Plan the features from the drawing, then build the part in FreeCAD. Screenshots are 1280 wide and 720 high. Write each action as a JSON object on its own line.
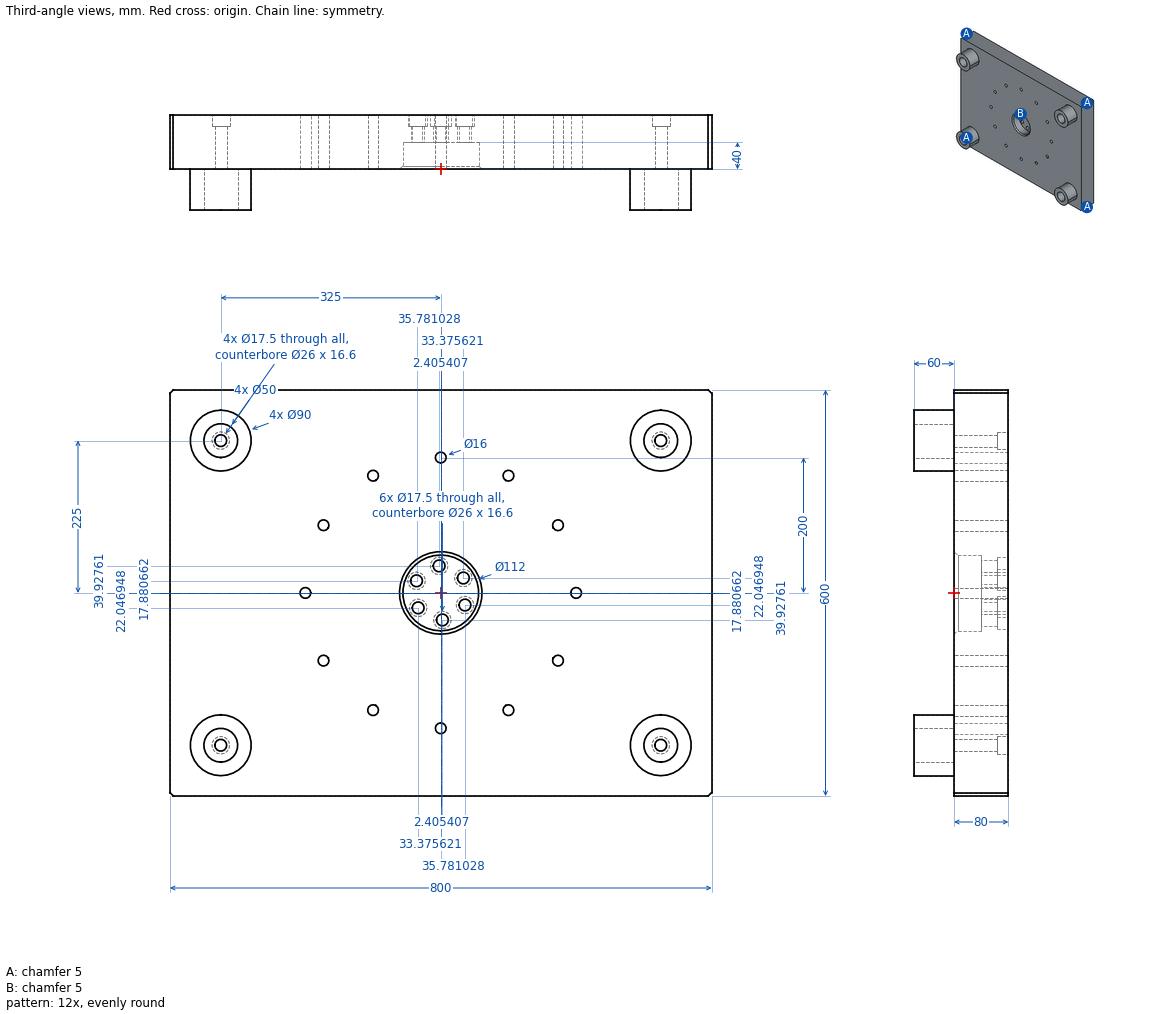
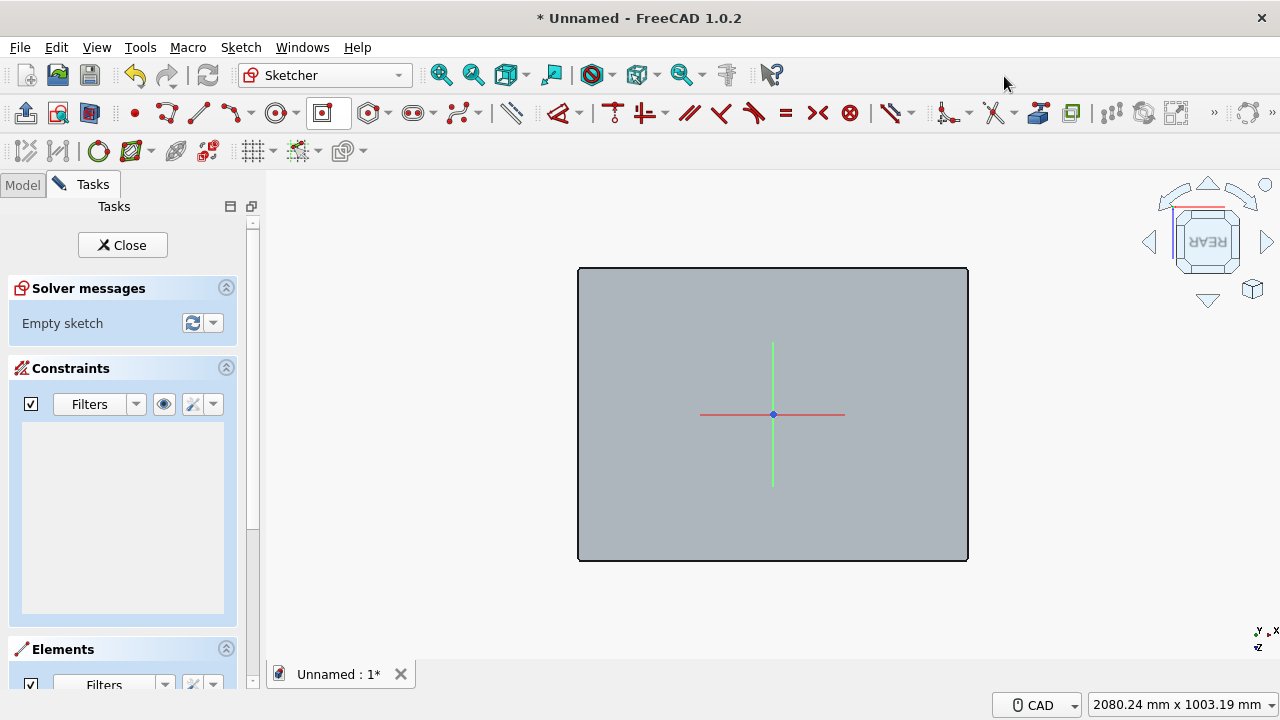
{"action": "scroll", "coordinate": [787, 415], "scroll_direction": "up", "scroll_amount": 9}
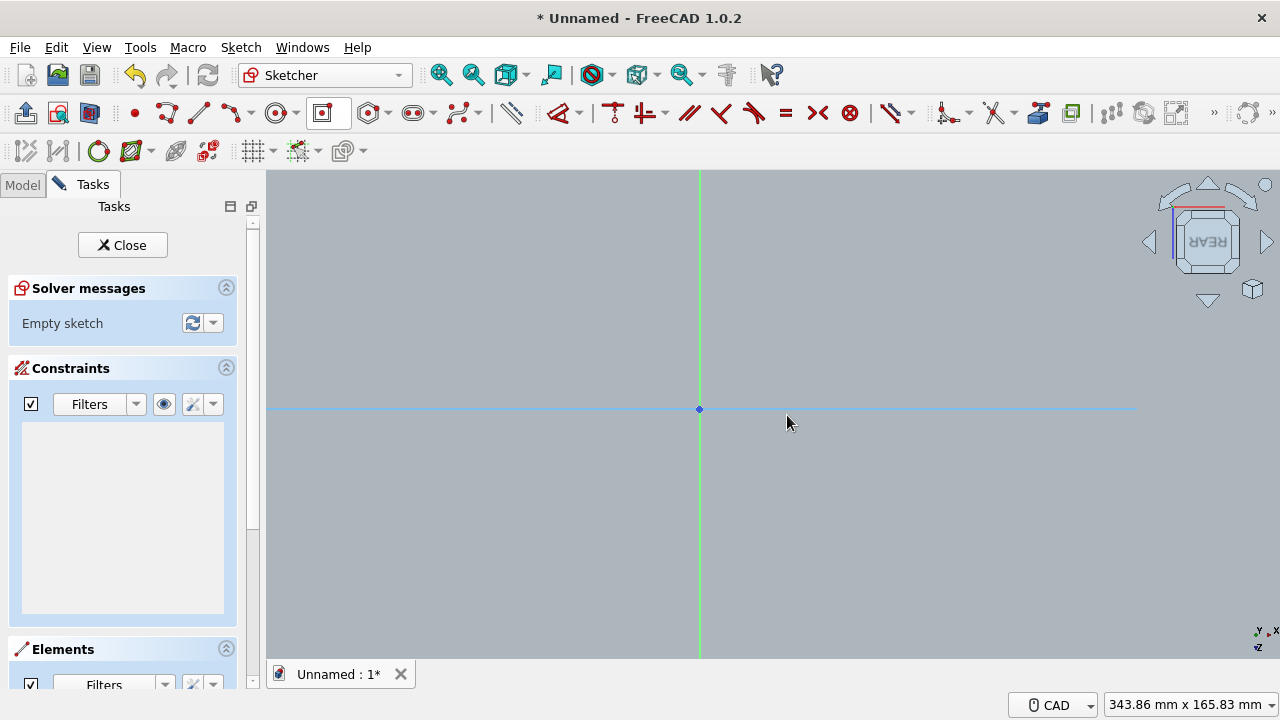
{"action": "left_click", "coordinate": [276, 114]}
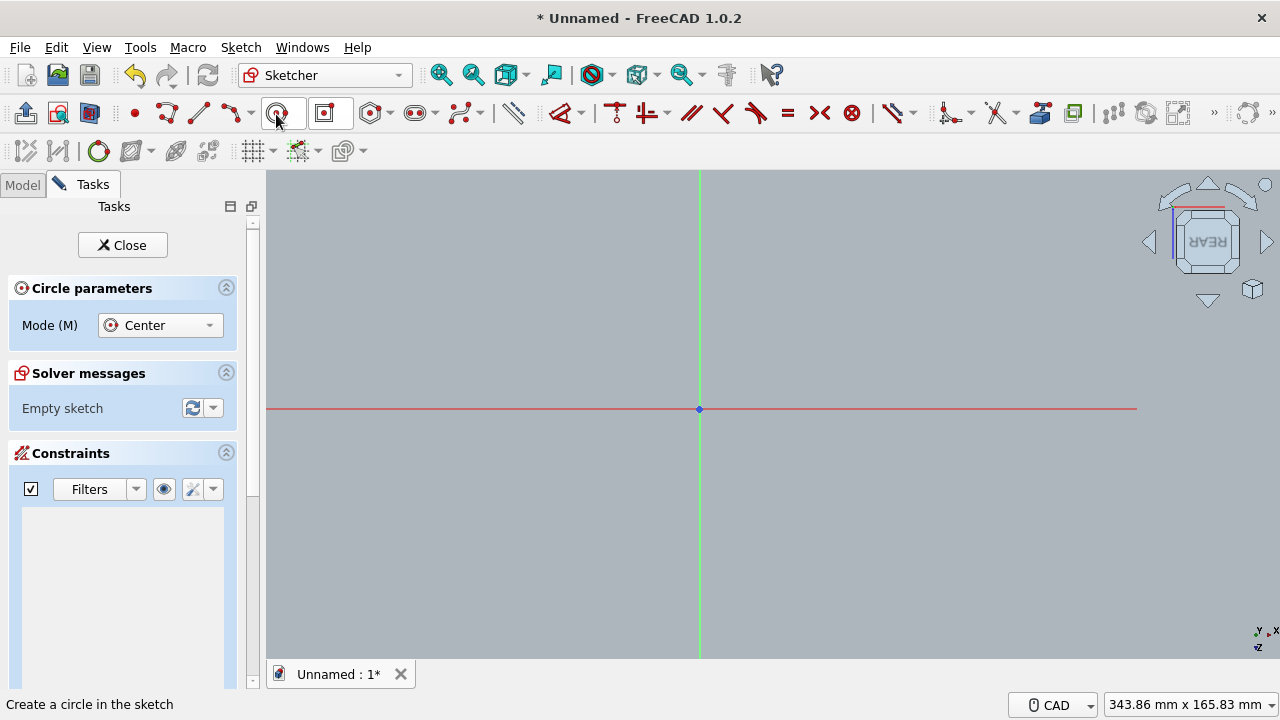
{"action": "scroll", "coordinate": [707, 292], "scroll_direction": "up", "scroll_amount": 5}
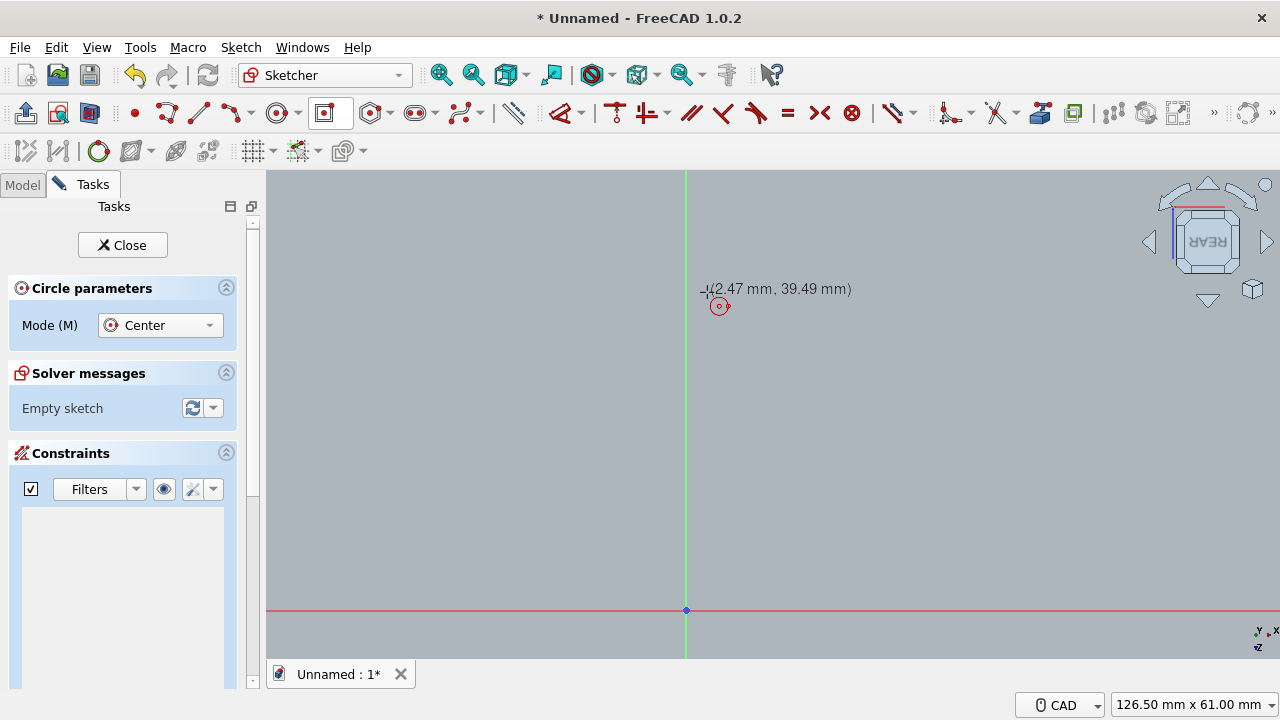
{"action": "left_click", "coordinate": [706, 291]}
{"action": "mouse_move", "coordinate": [755, 241]}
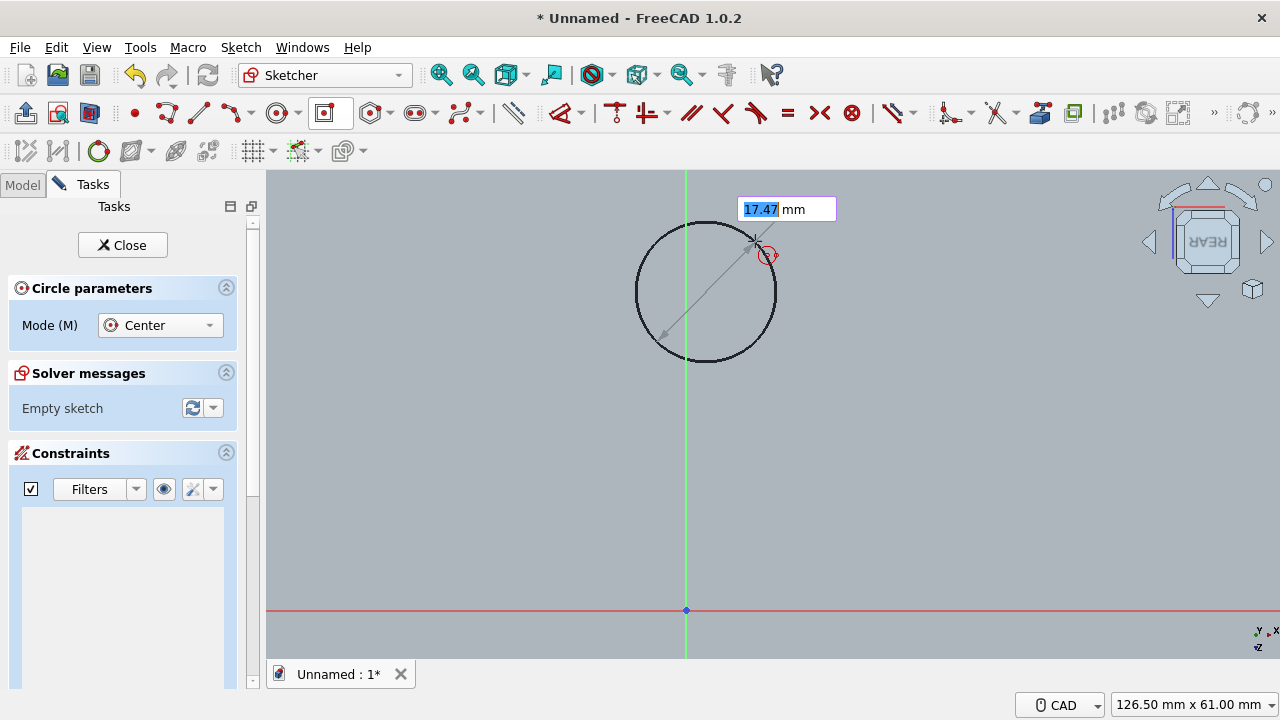
{"action": "type", "text": "17.5"}
{"action": "key", "text": "Return"}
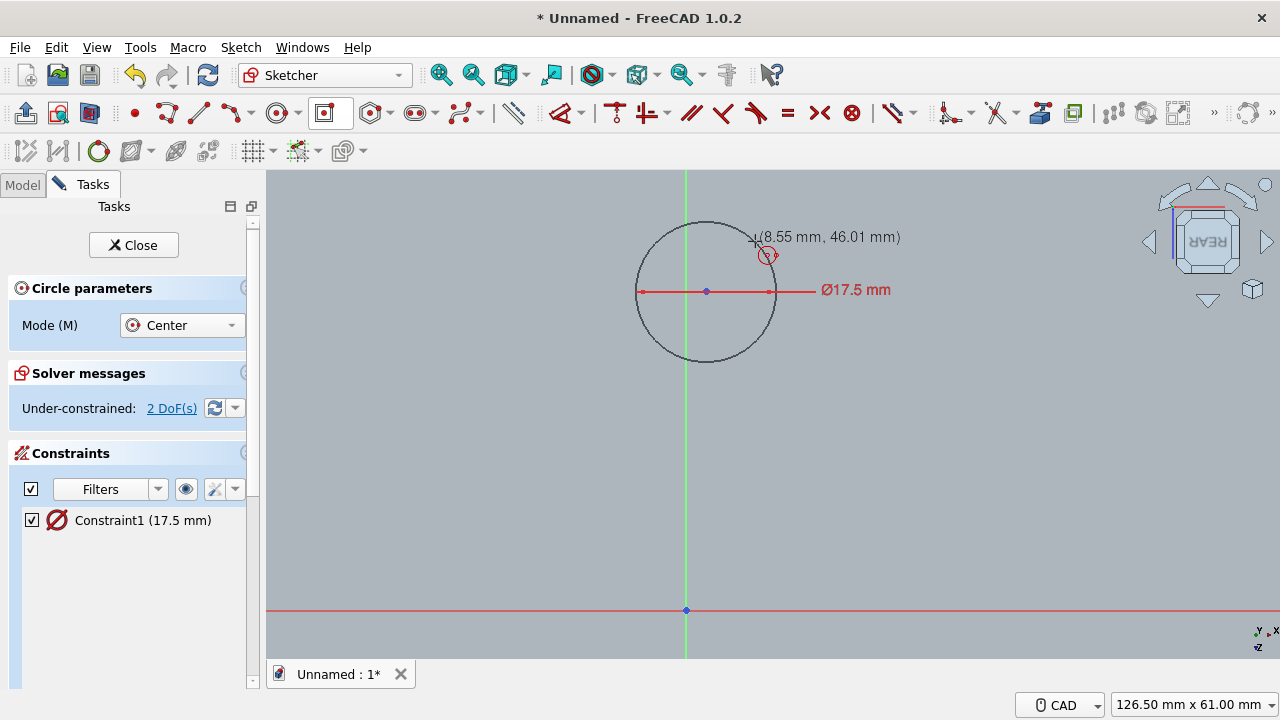
{"action": "left_click", "coordinate": [973, 467]}
{"action": "mouse_move", "coordinate": [1023, 418]}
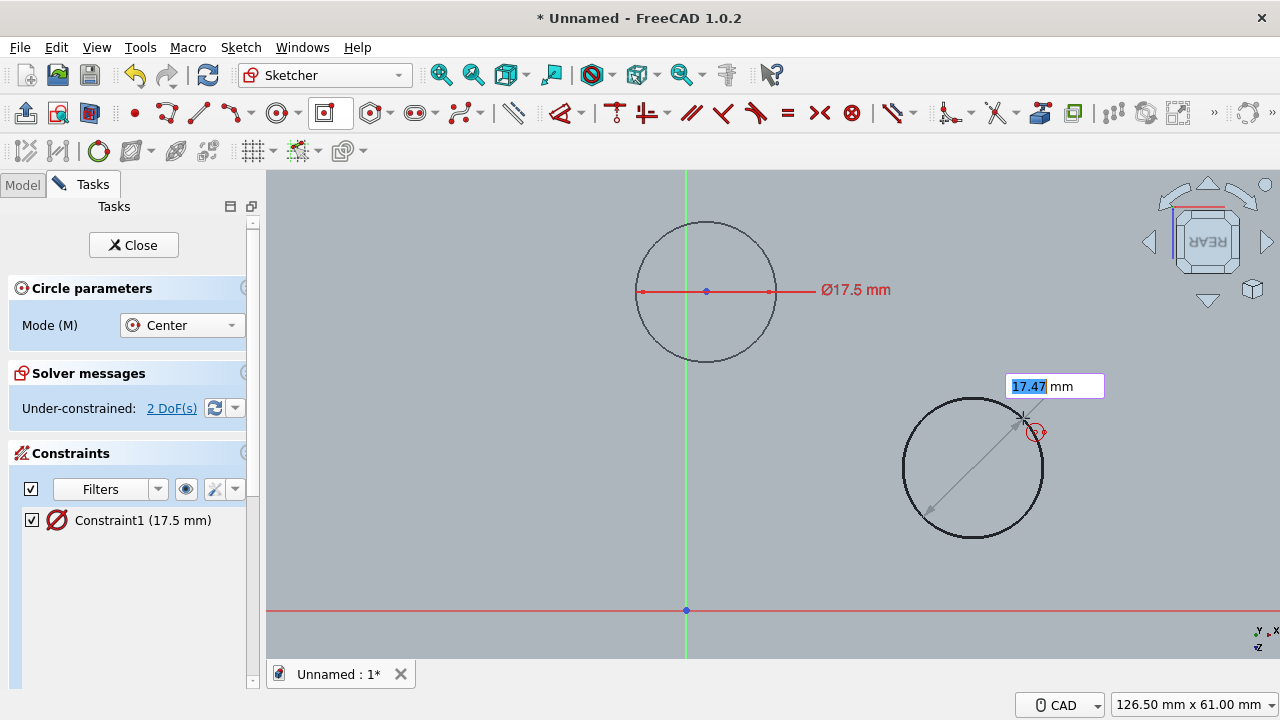
{"action": "type", "text": "17.5"}
{"action": "key", "text": "Return"}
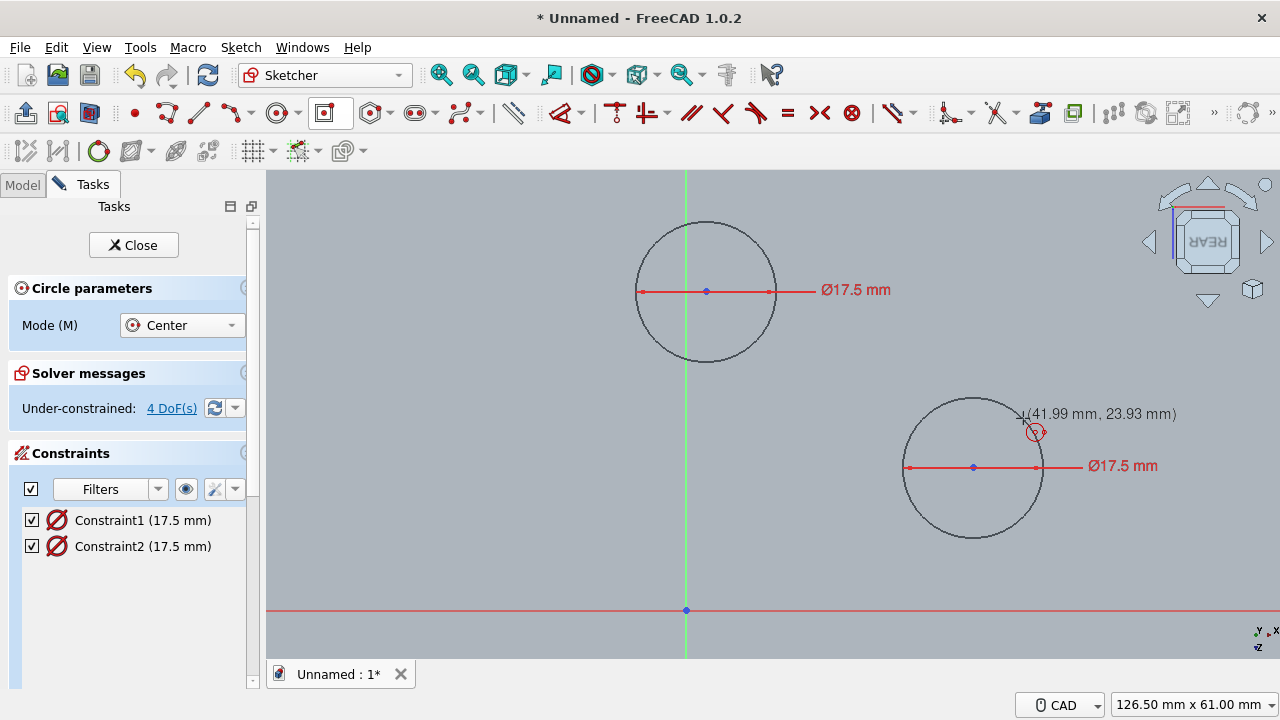
{"action": "scroll", "coordinate": [715, 300], "scroll_direction": "down", "scroll_amount": 5}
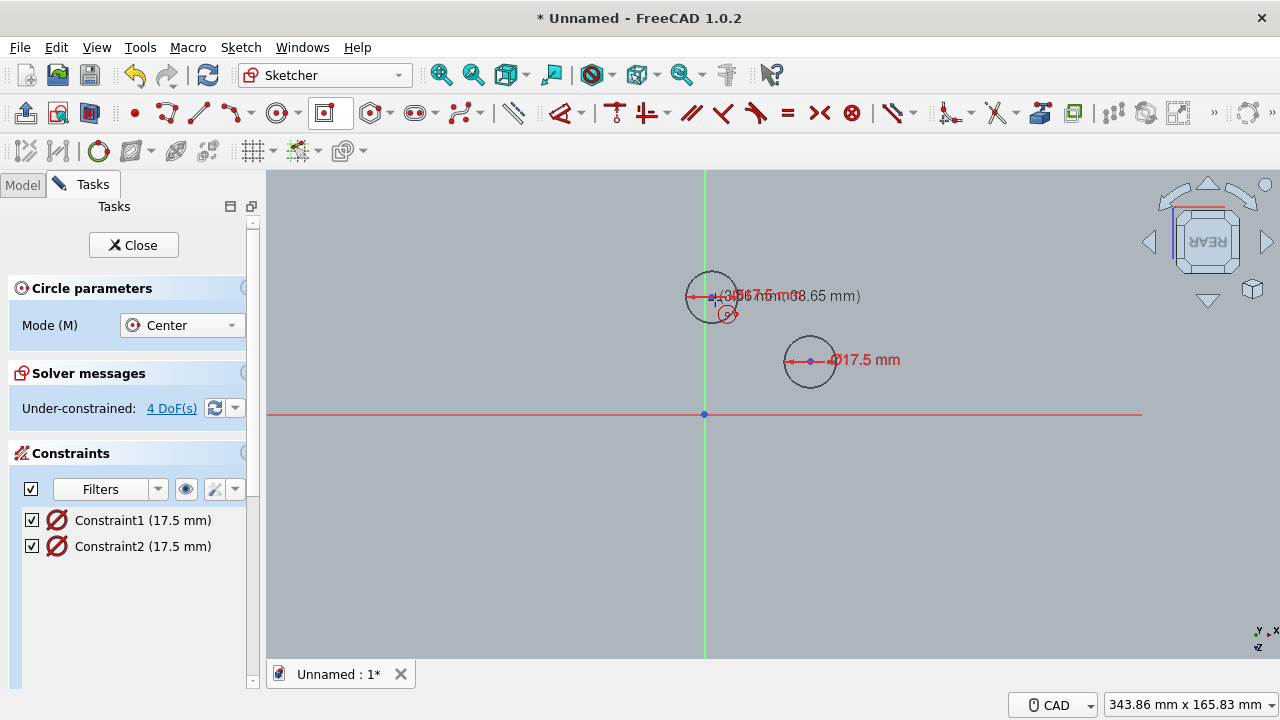
{"action": "left_click", "coordinate": [803, 480]}
{"action": "mouse_move", "coordinate": [821, 461]}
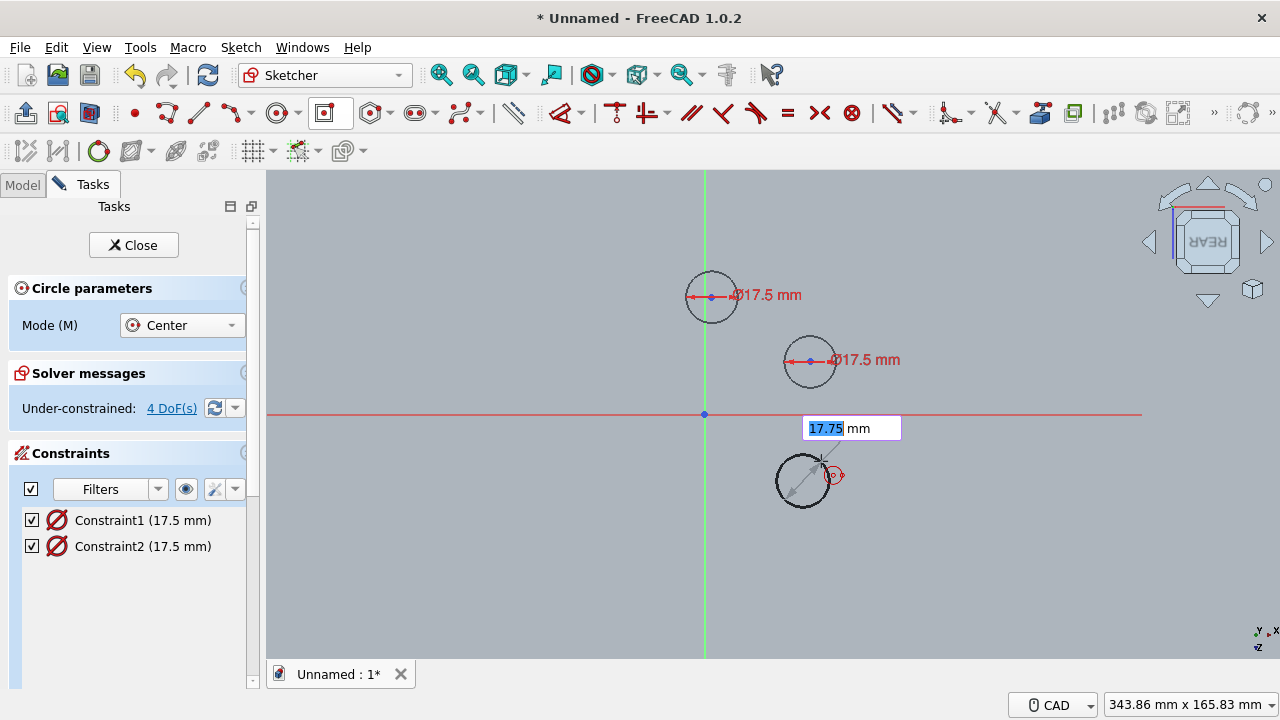
{"action": "type", "text": "17.5"}
{"action": "key", "text": "Return"}